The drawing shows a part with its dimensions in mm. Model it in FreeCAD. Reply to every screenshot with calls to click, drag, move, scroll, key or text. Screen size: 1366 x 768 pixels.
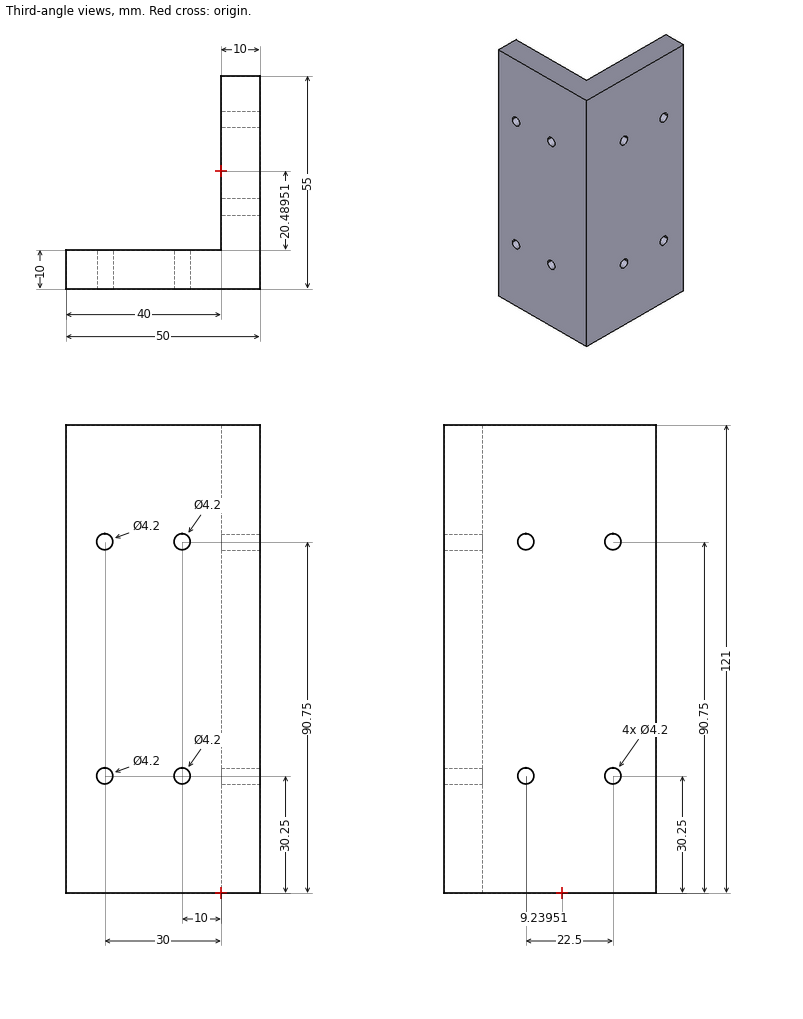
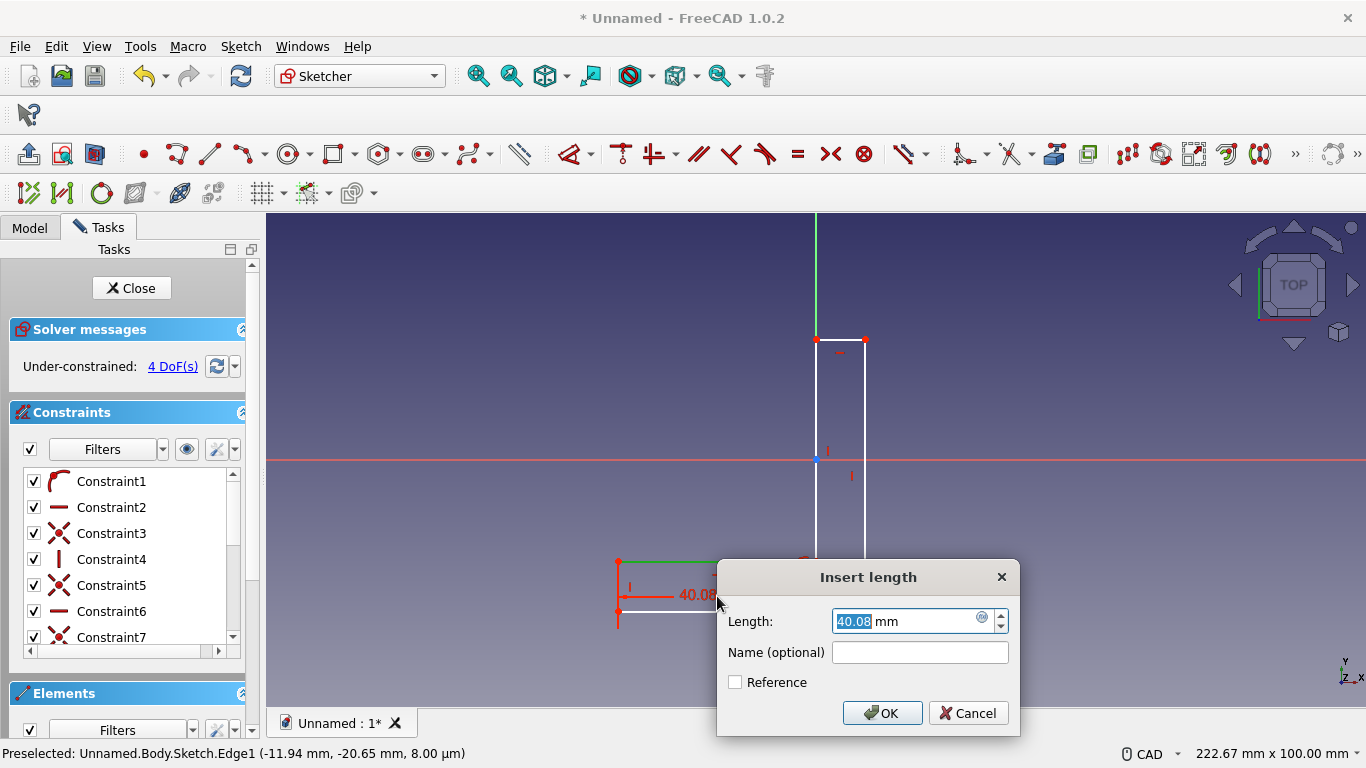
text(40)
key(Return)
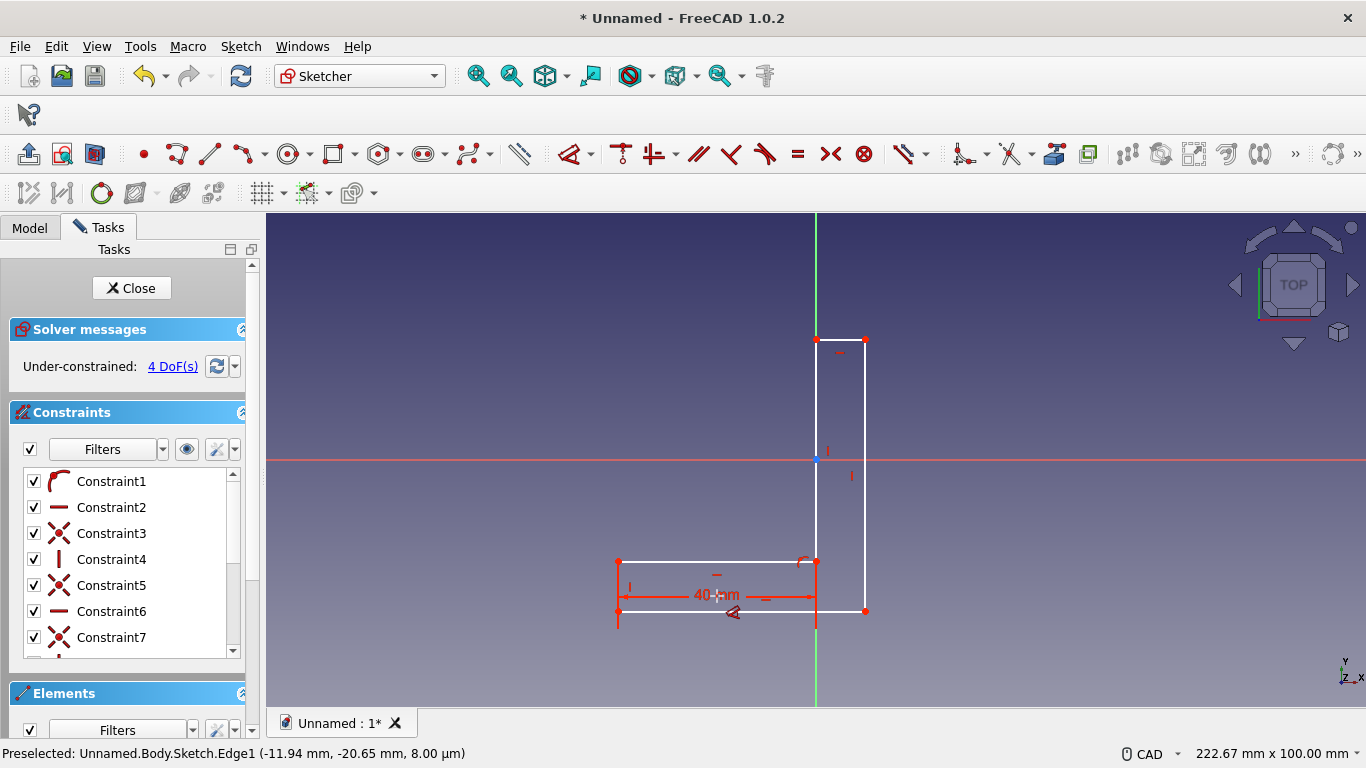
click(618, 577)
click(584, 587)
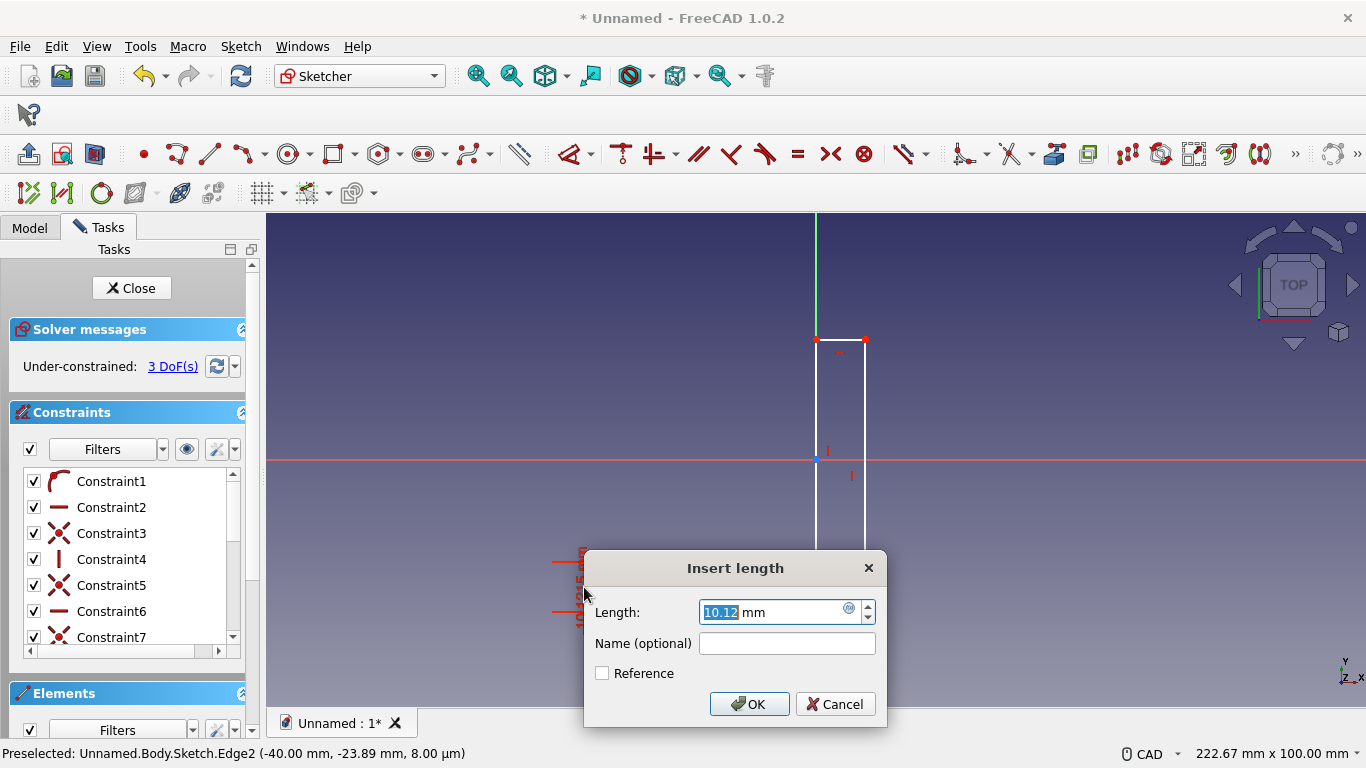
text(10)
key(Return)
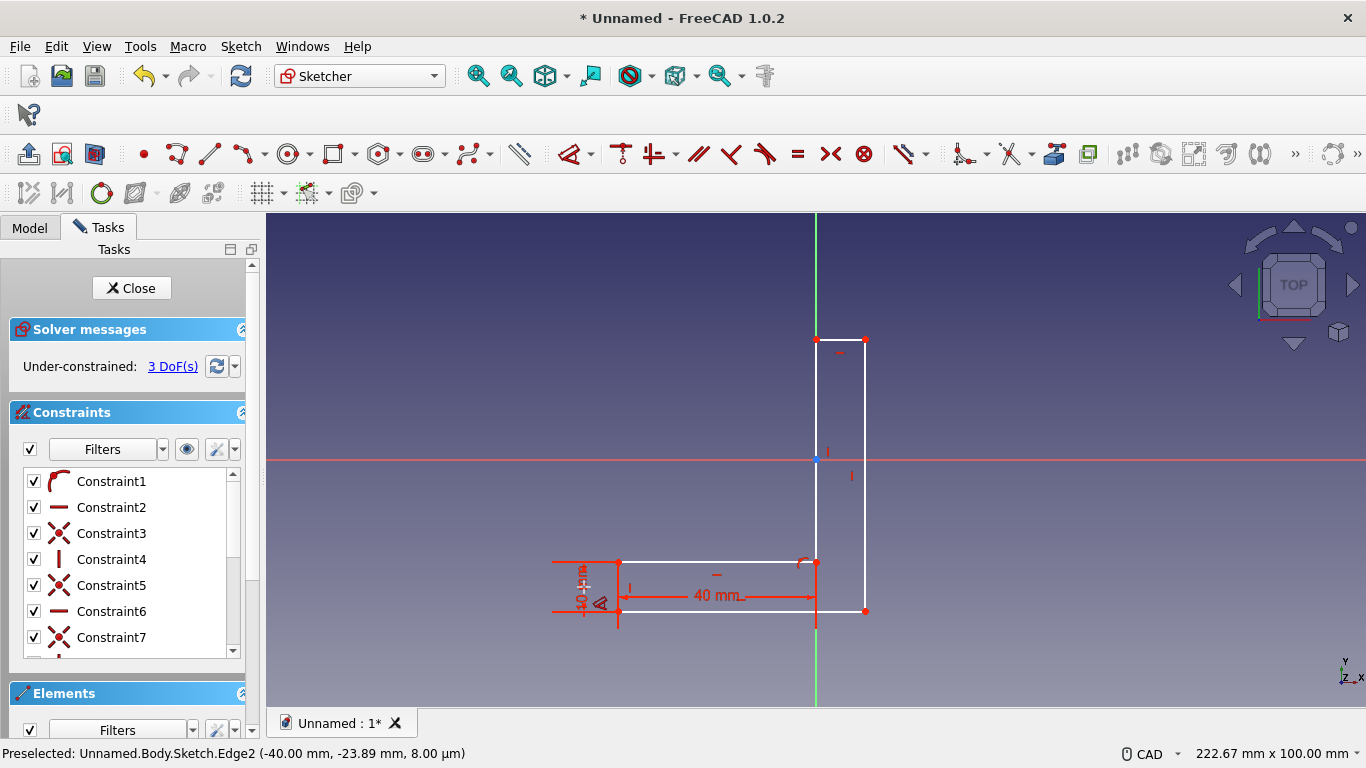
click(692, 612)
click(742, 646)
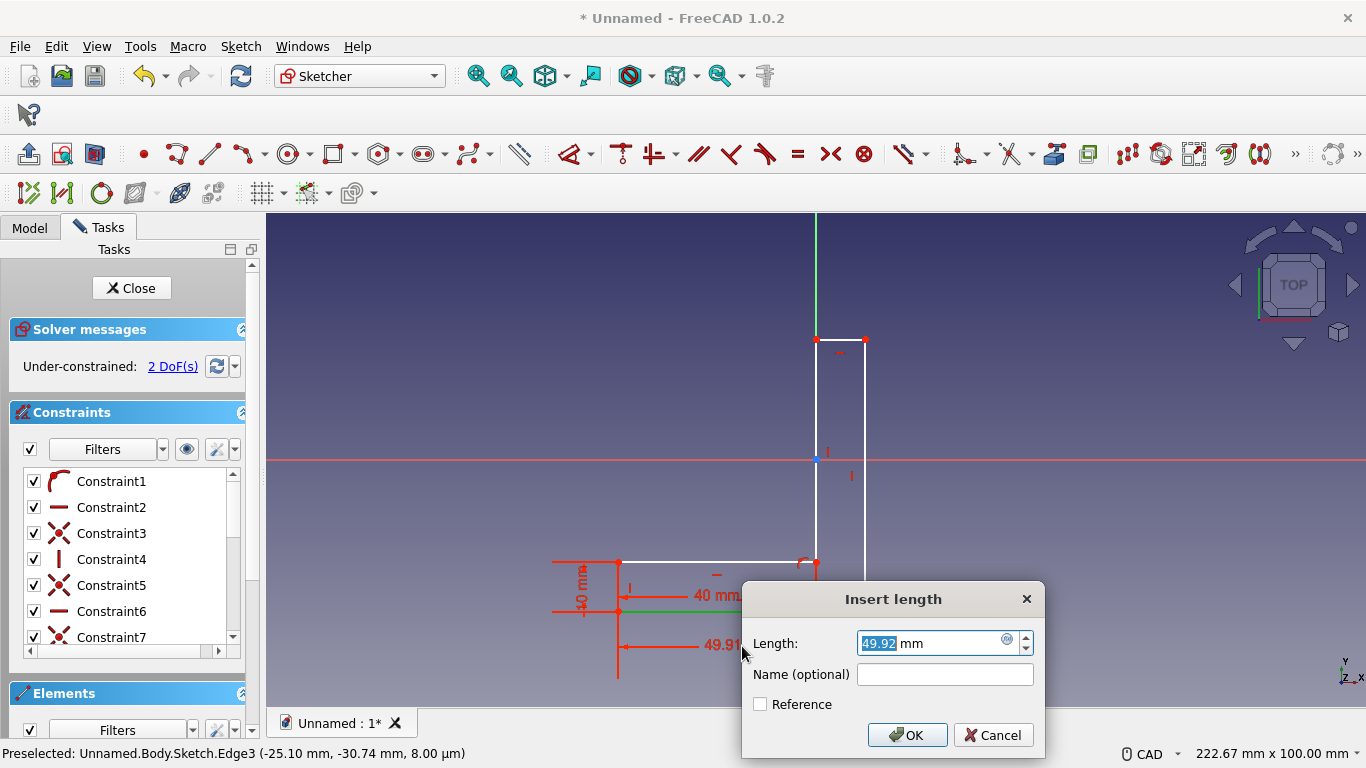
text(50)
key(Return)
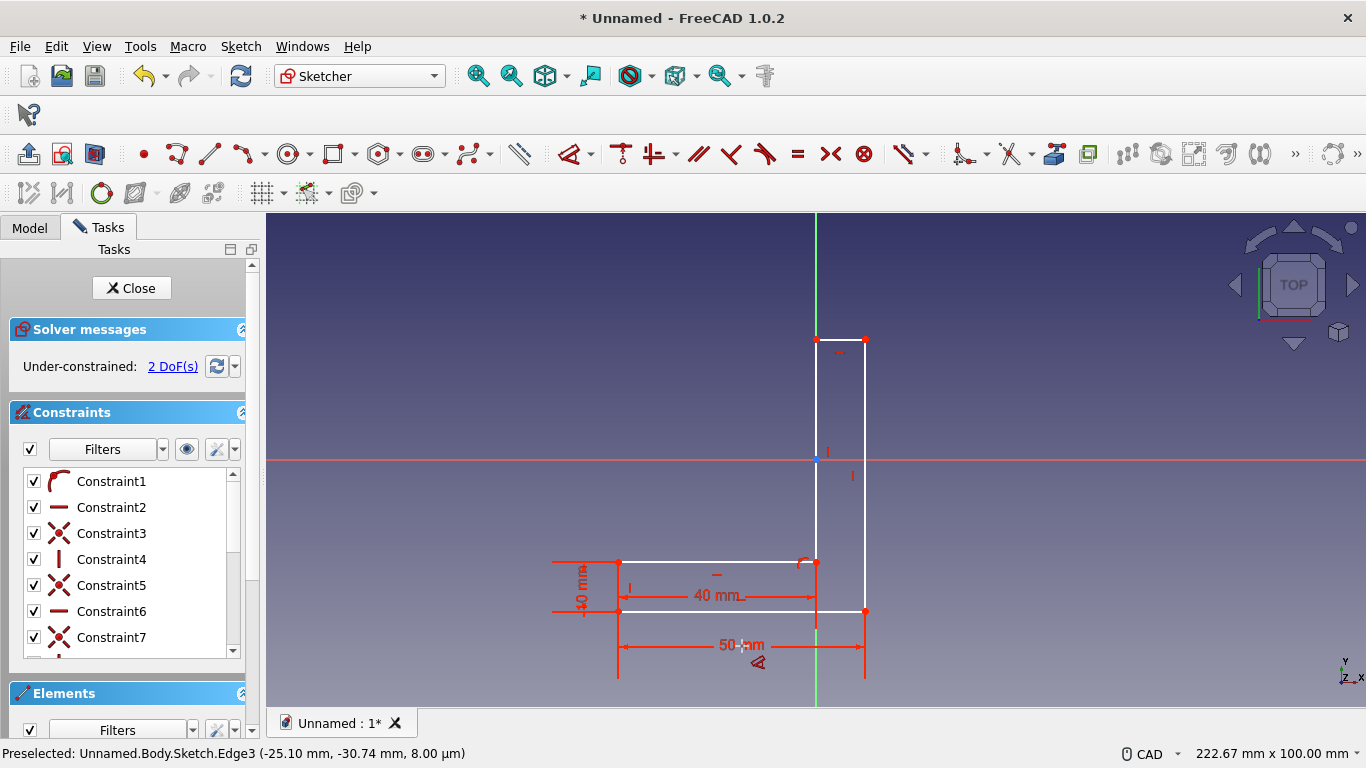
click(865, 530)
click(899, 476)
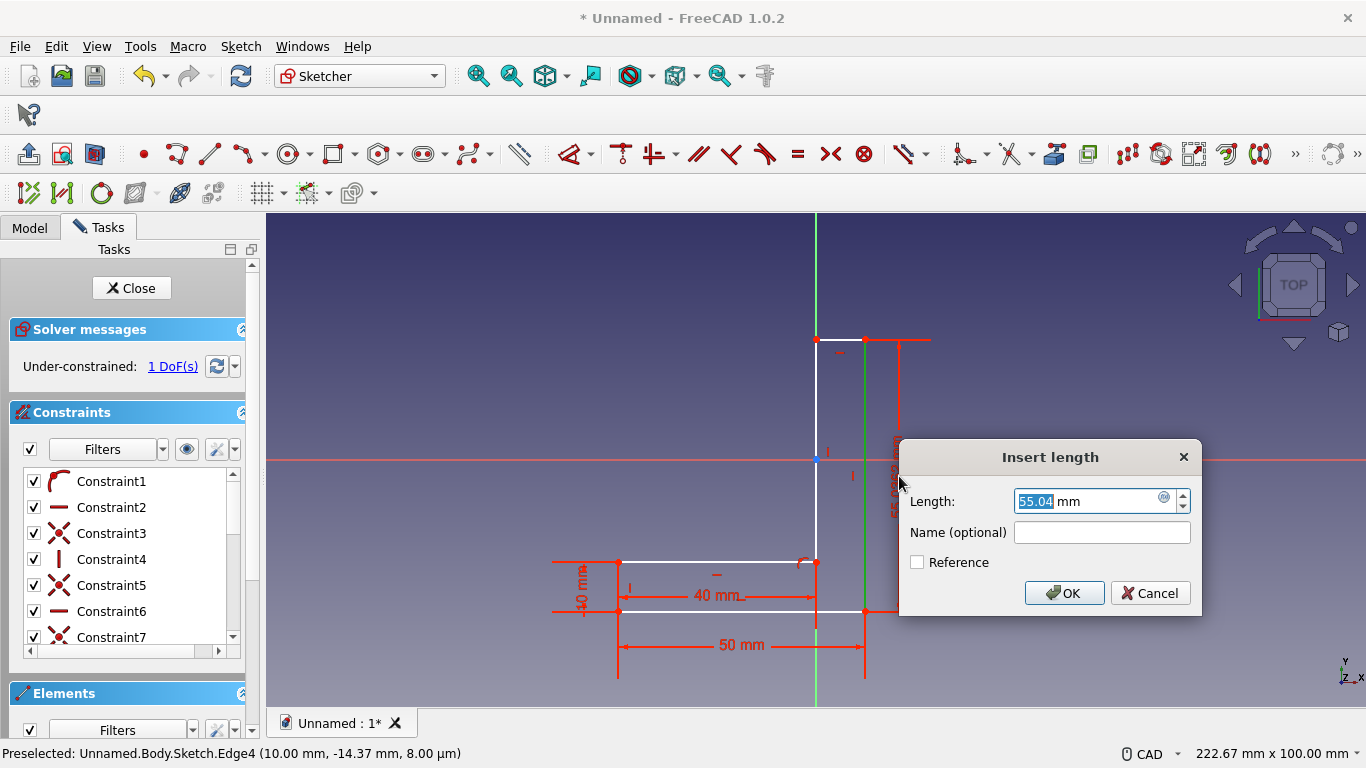
text(55)
key(Return)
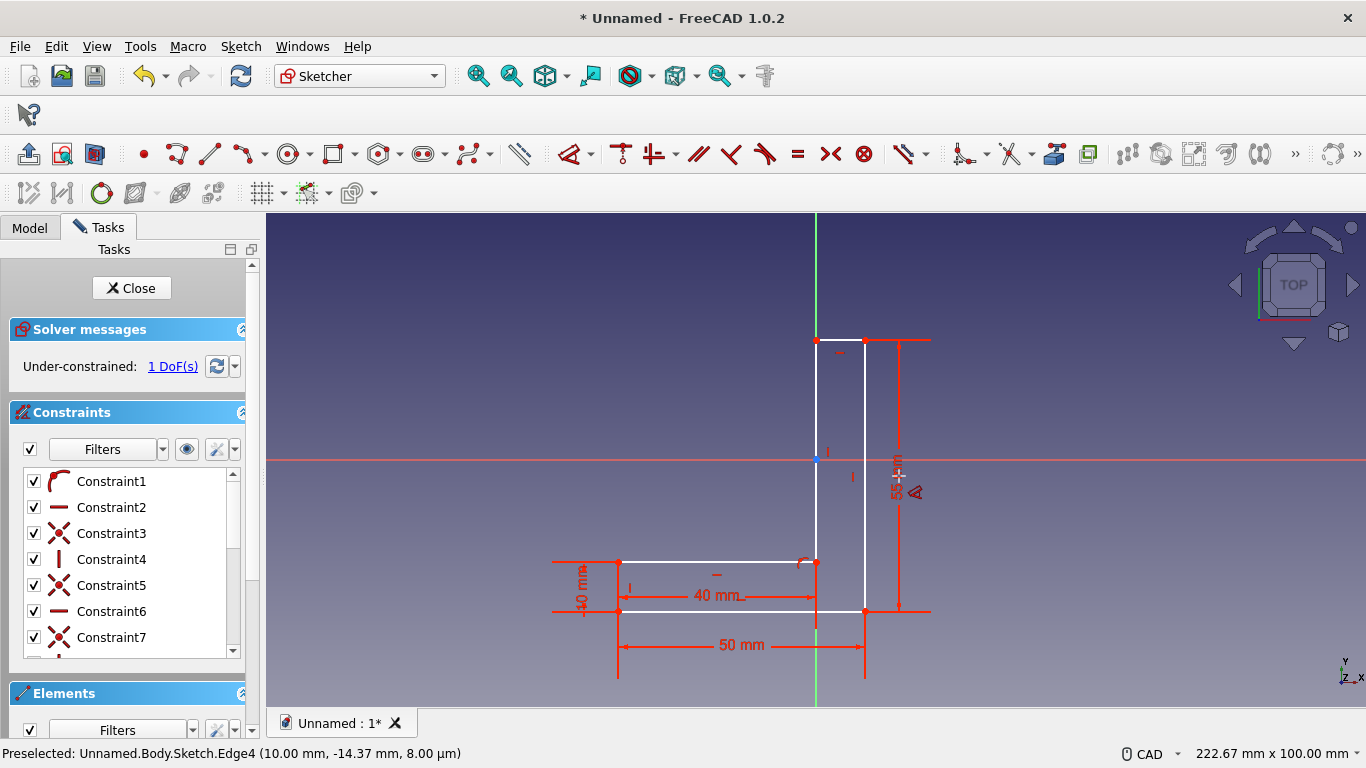
click(816, 562)
click(850, 511)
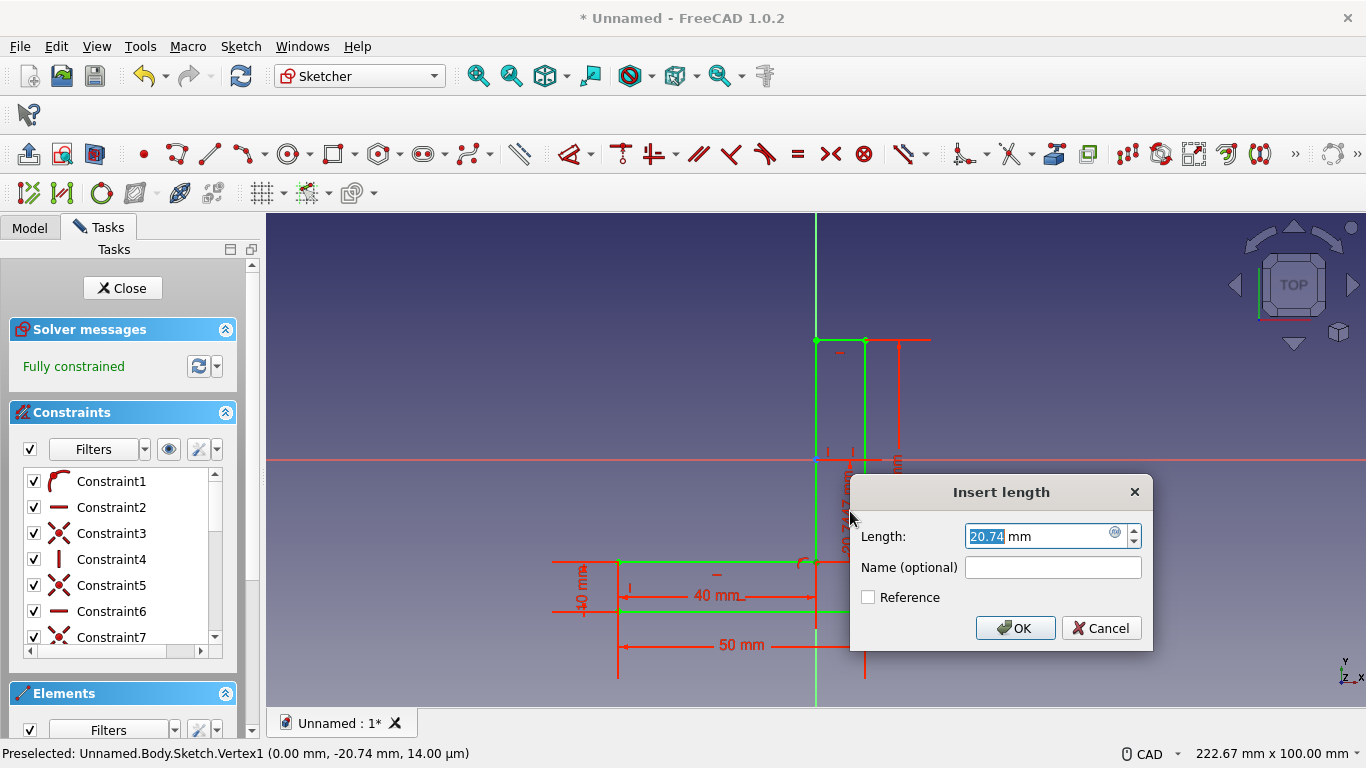
text(20.48951)
key(Return)
key(Escape)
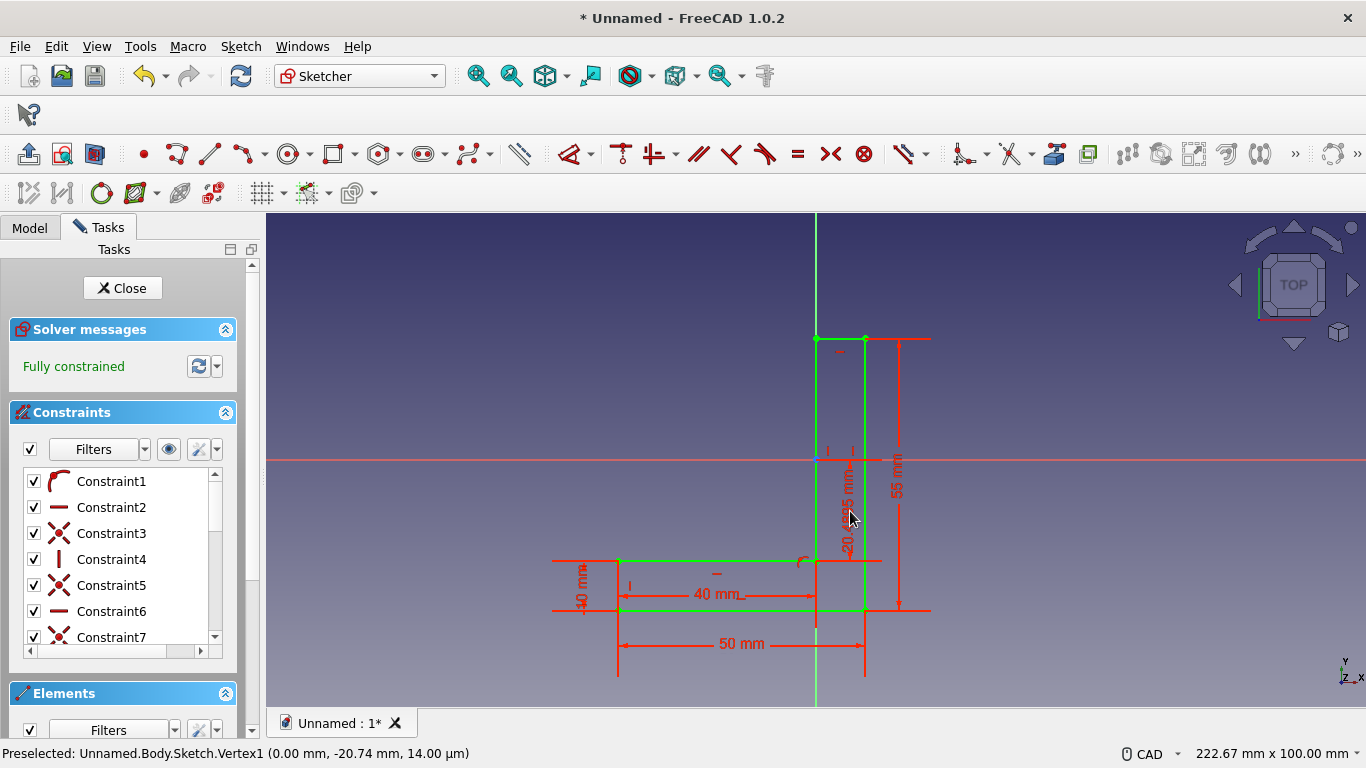
click(123, 288)